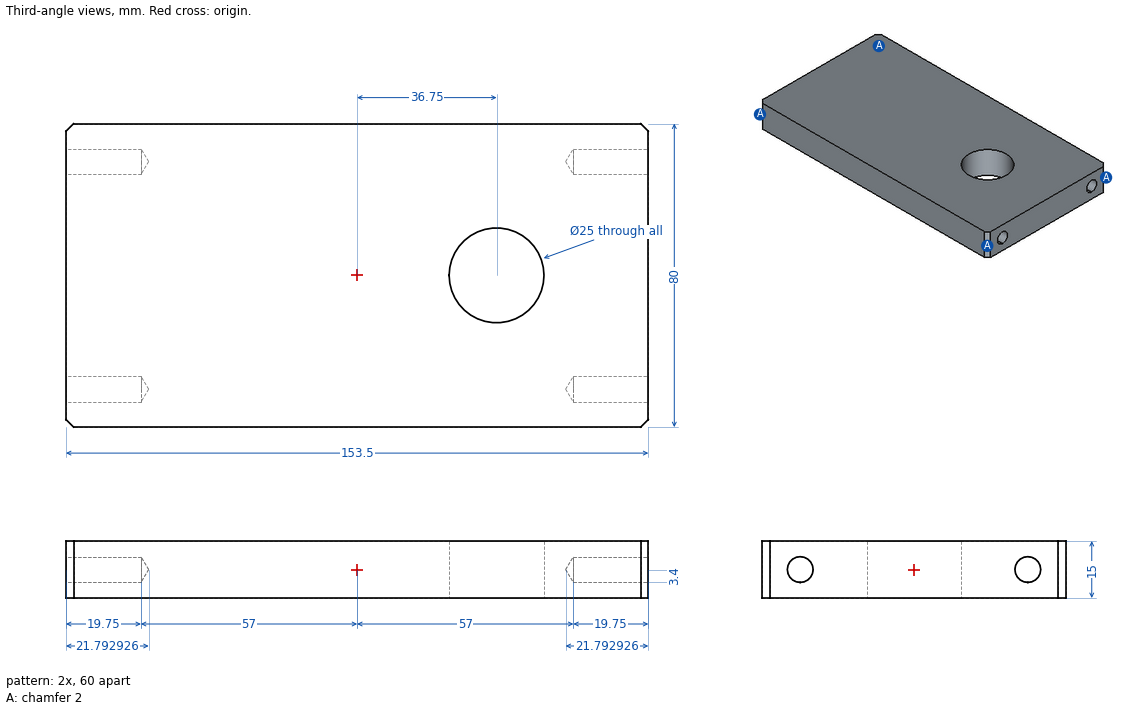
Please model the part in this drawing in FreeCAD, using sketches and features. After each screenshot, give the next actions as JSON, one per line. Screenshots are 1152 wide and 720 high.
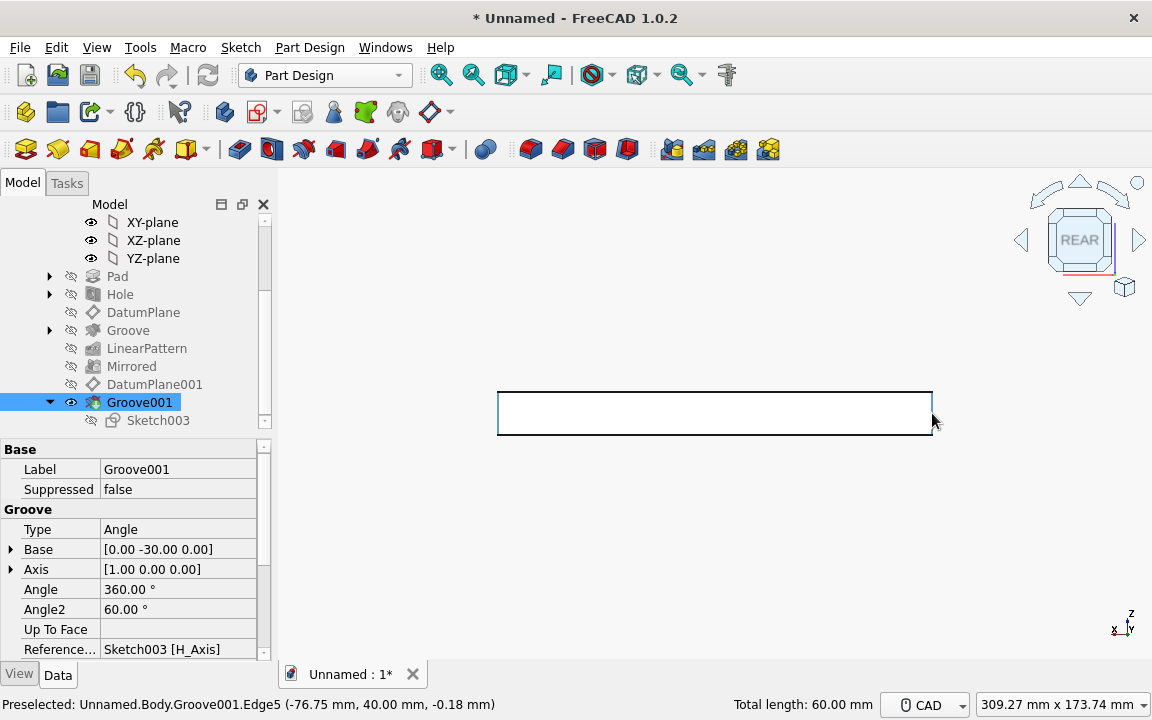
{"action": "left_click", "coordinate": [564, 150]}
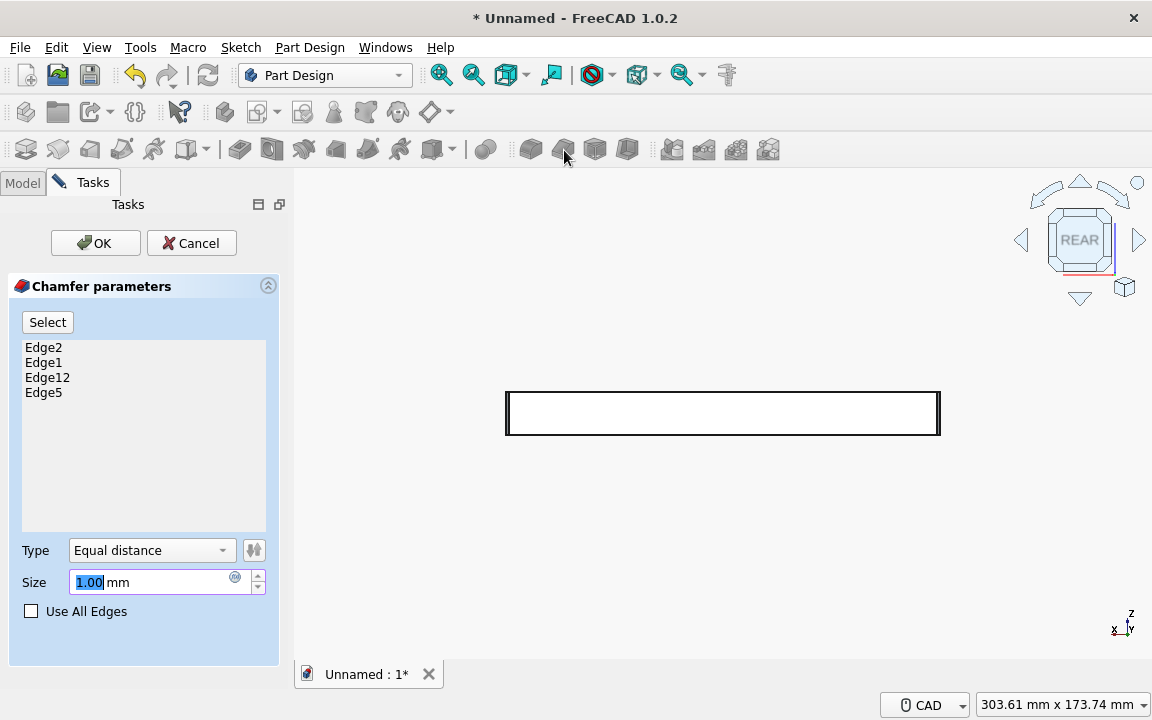
{"action": "type", "text": "2"}
{"action": "key", "text": "Tab"}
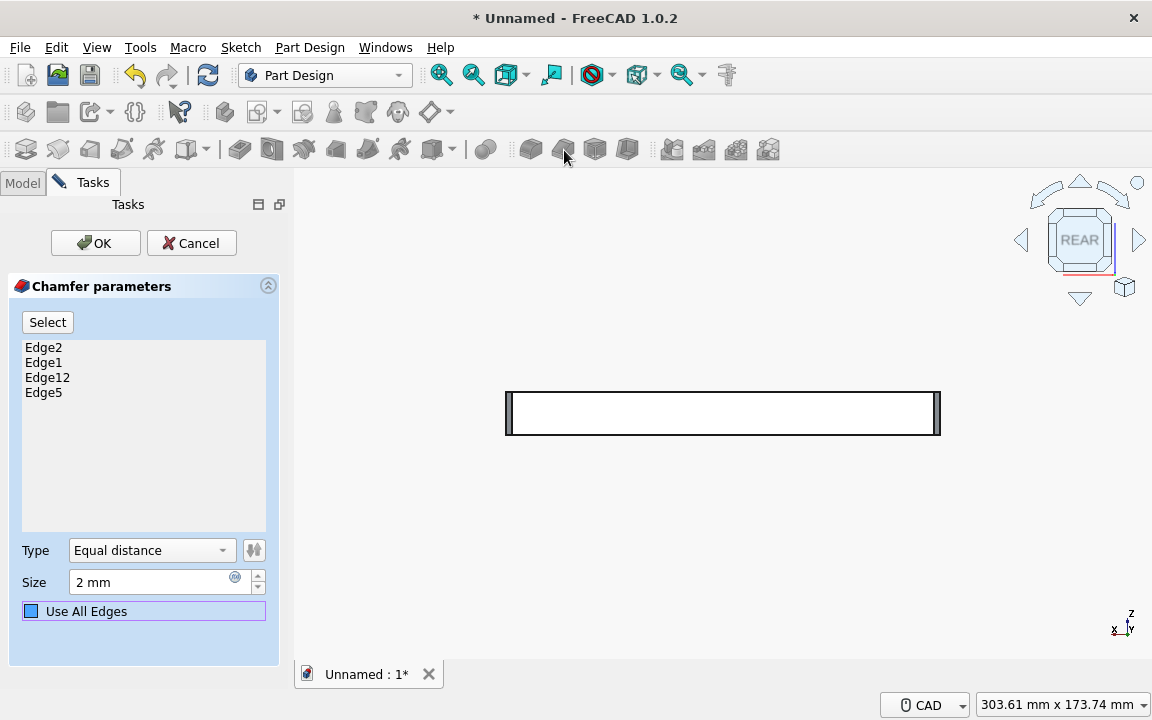
{"action": "left_click", "coordinate": [96, 243]}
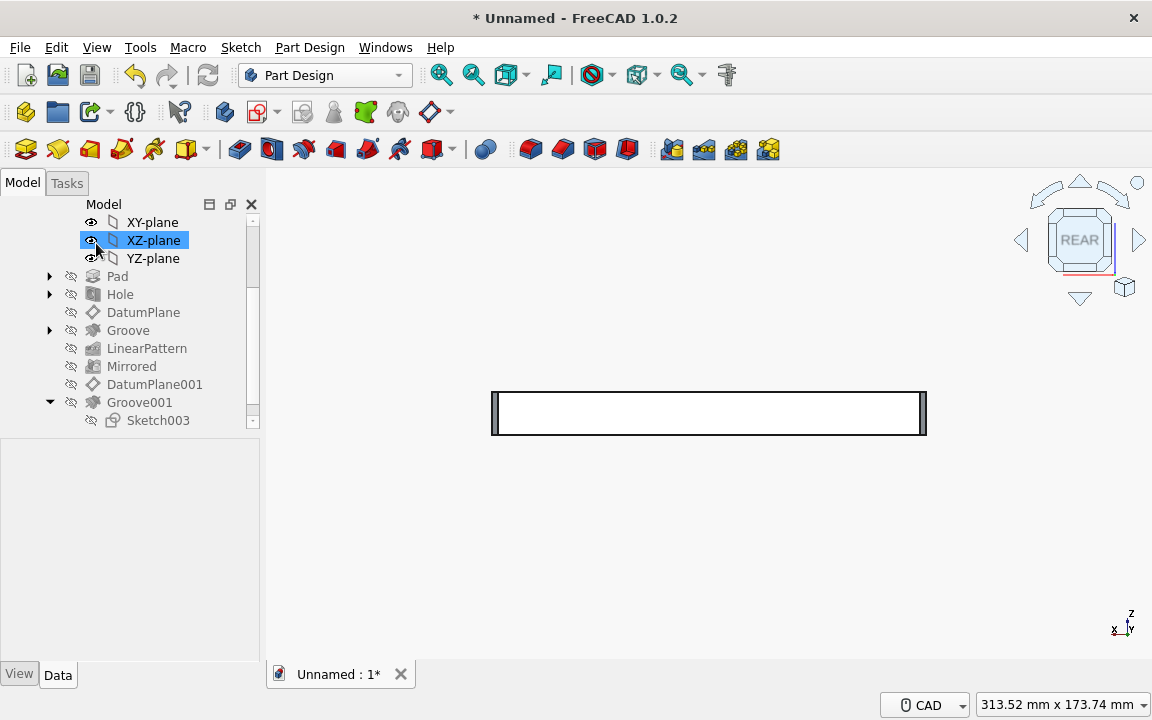
{"action": "key", "text": "0"}